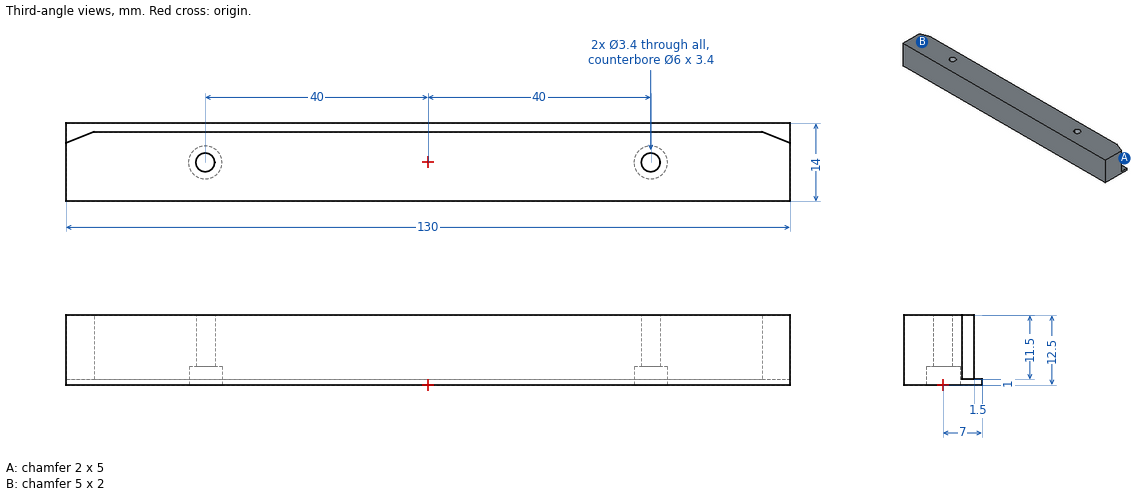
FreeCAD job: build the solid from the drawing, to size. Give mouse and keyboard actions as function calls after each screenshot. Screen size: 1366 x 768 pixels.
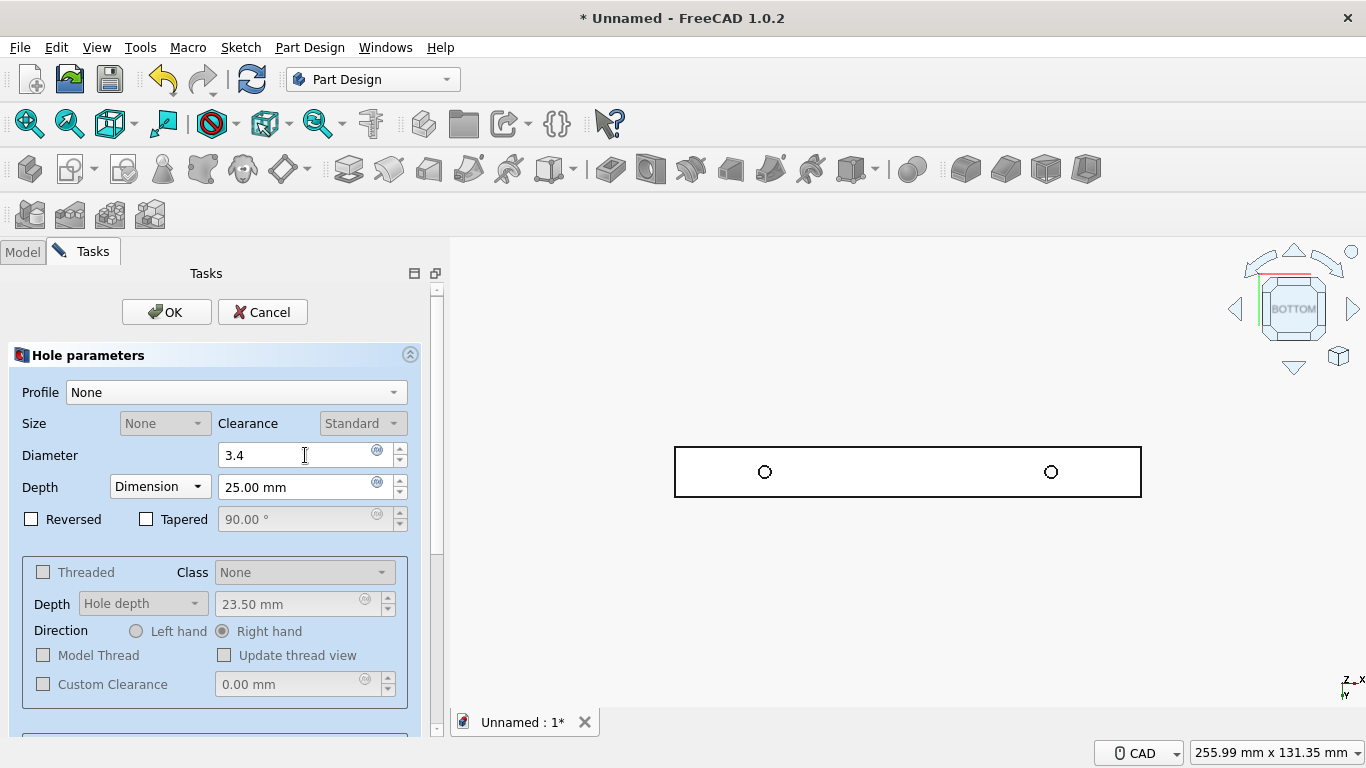
click(161, 486)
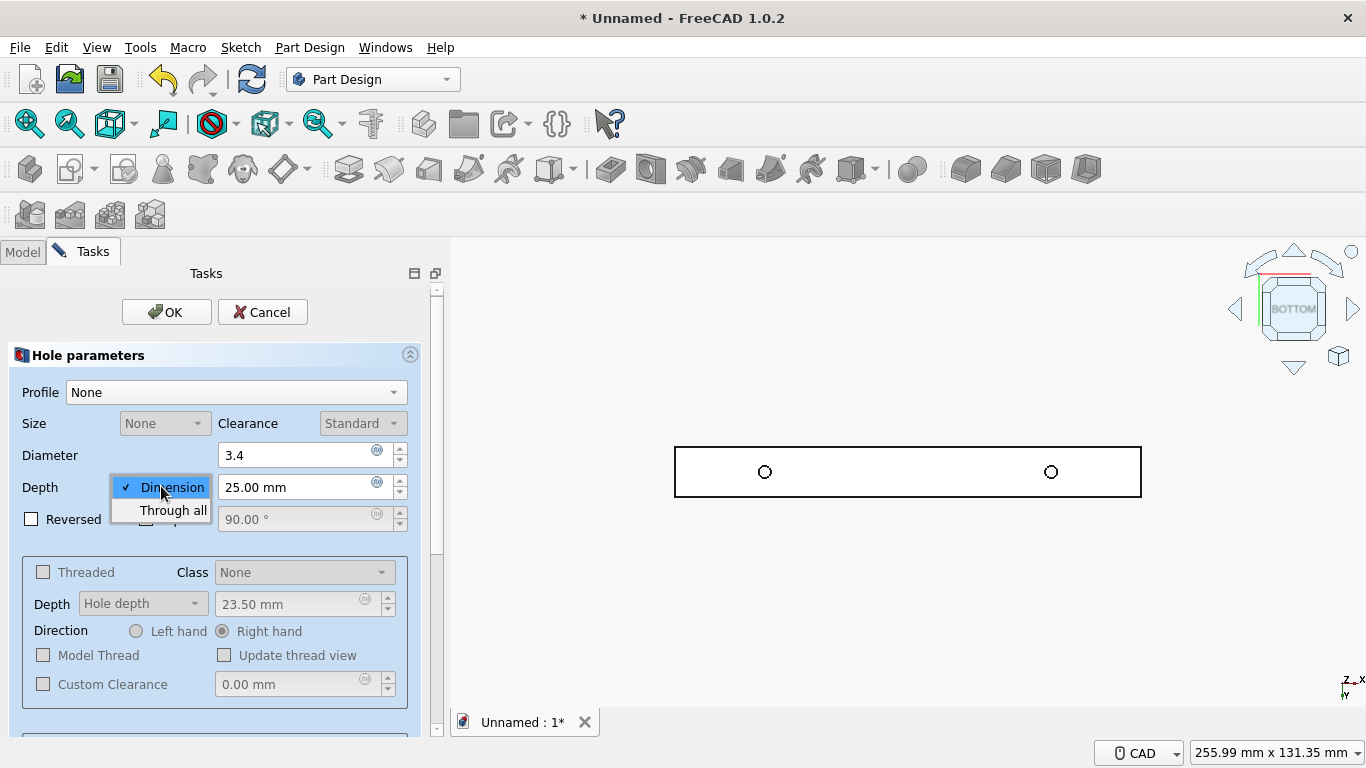
click(160, 510)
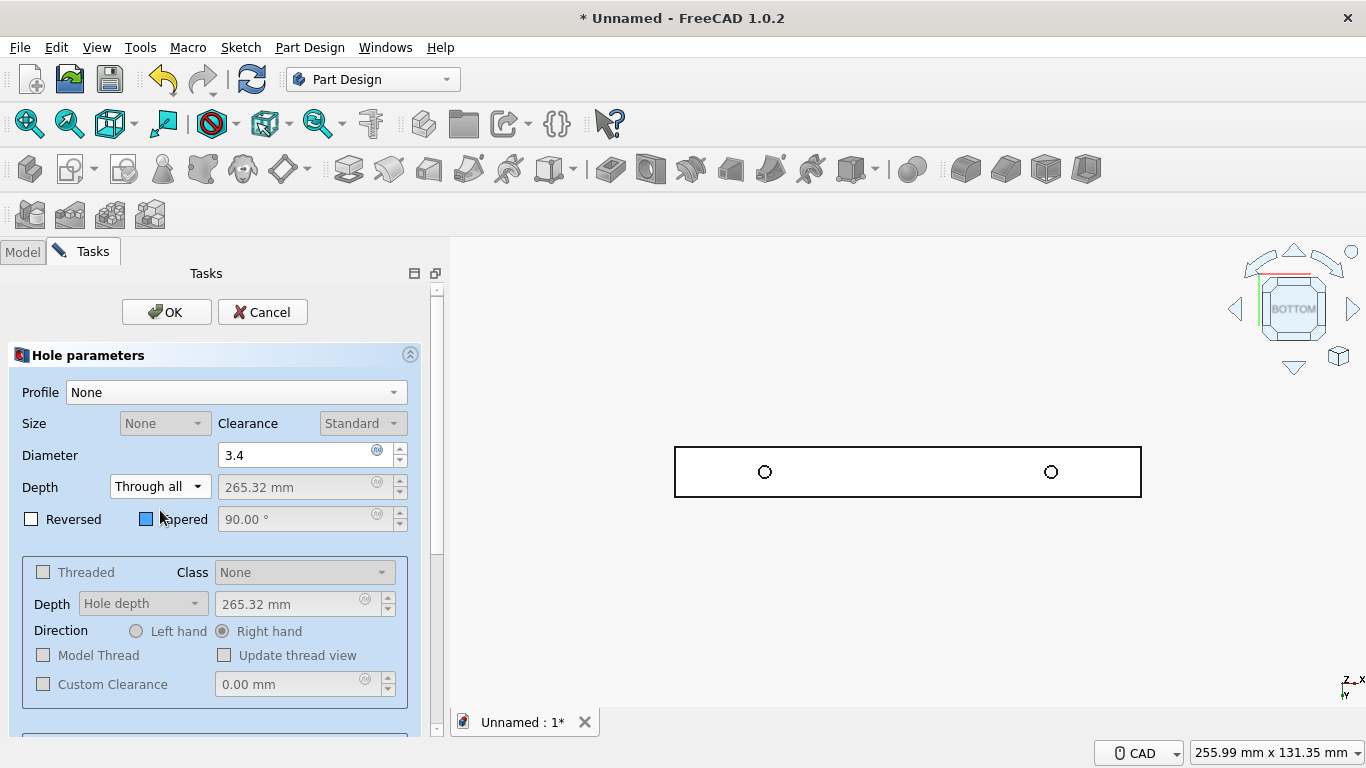
scroll(437, 510, down, 2)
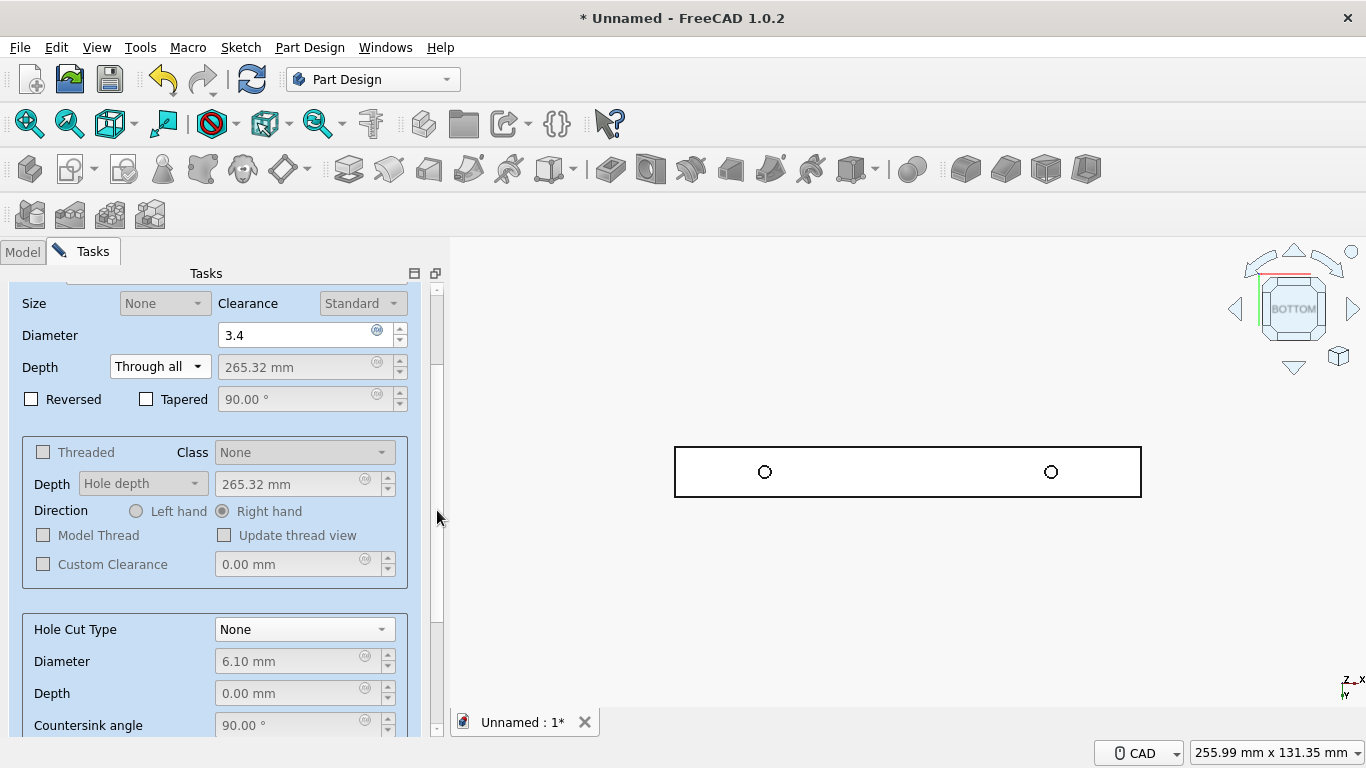
click(306, 630)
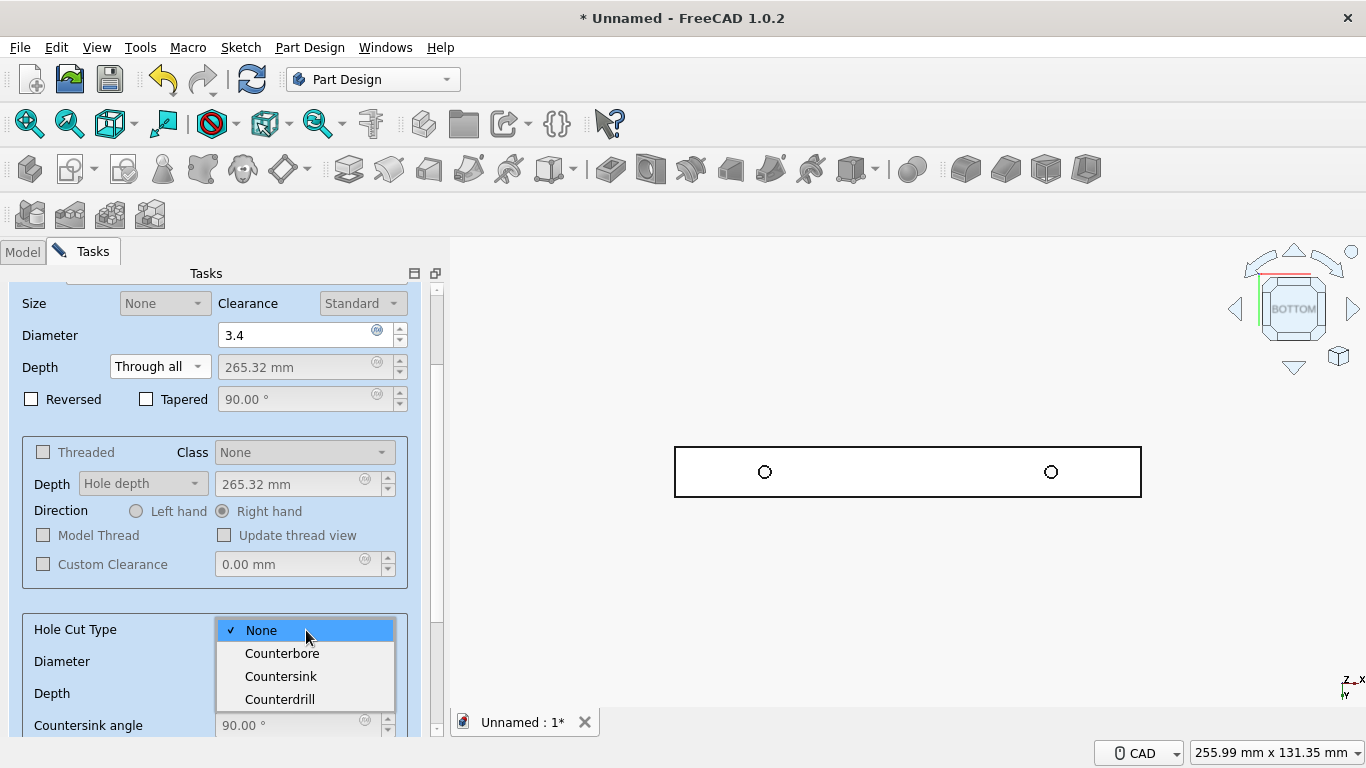
click(304, 654)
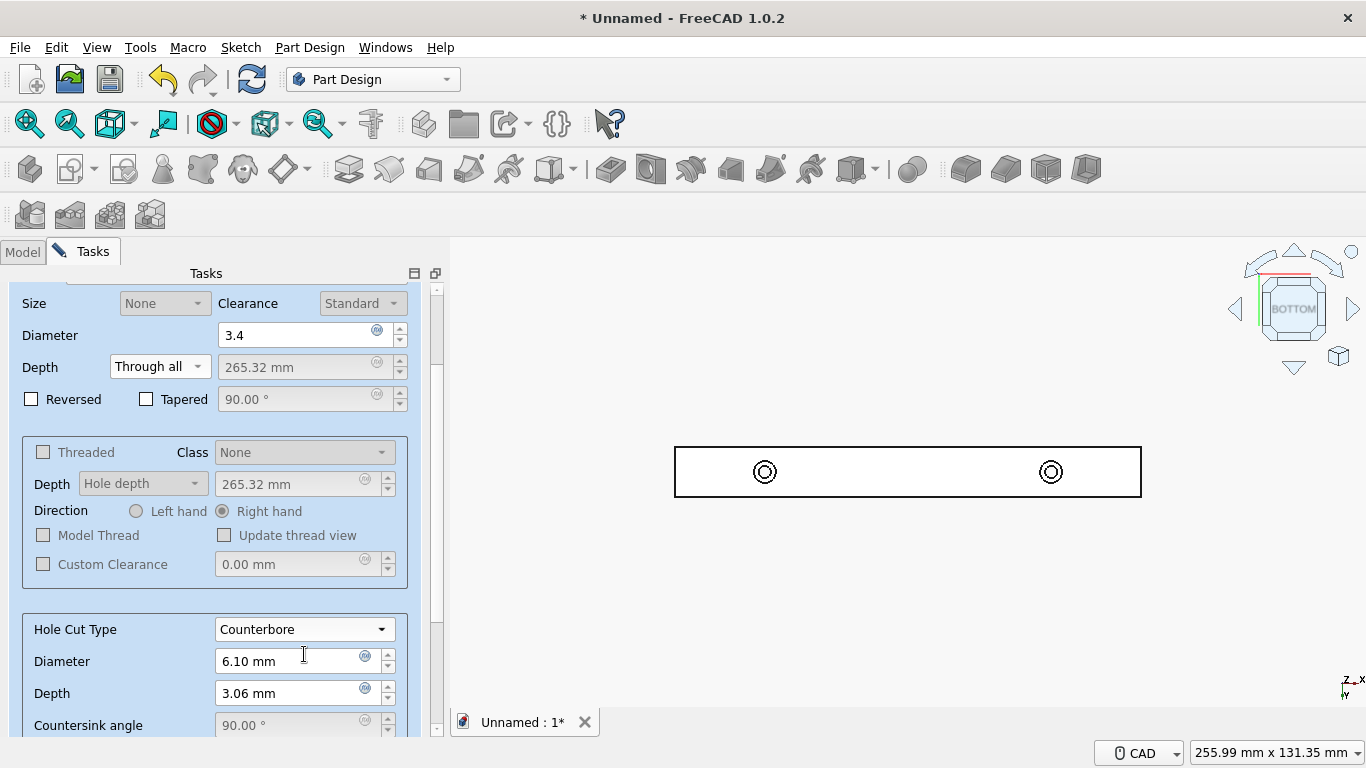
triple_click(298, 661)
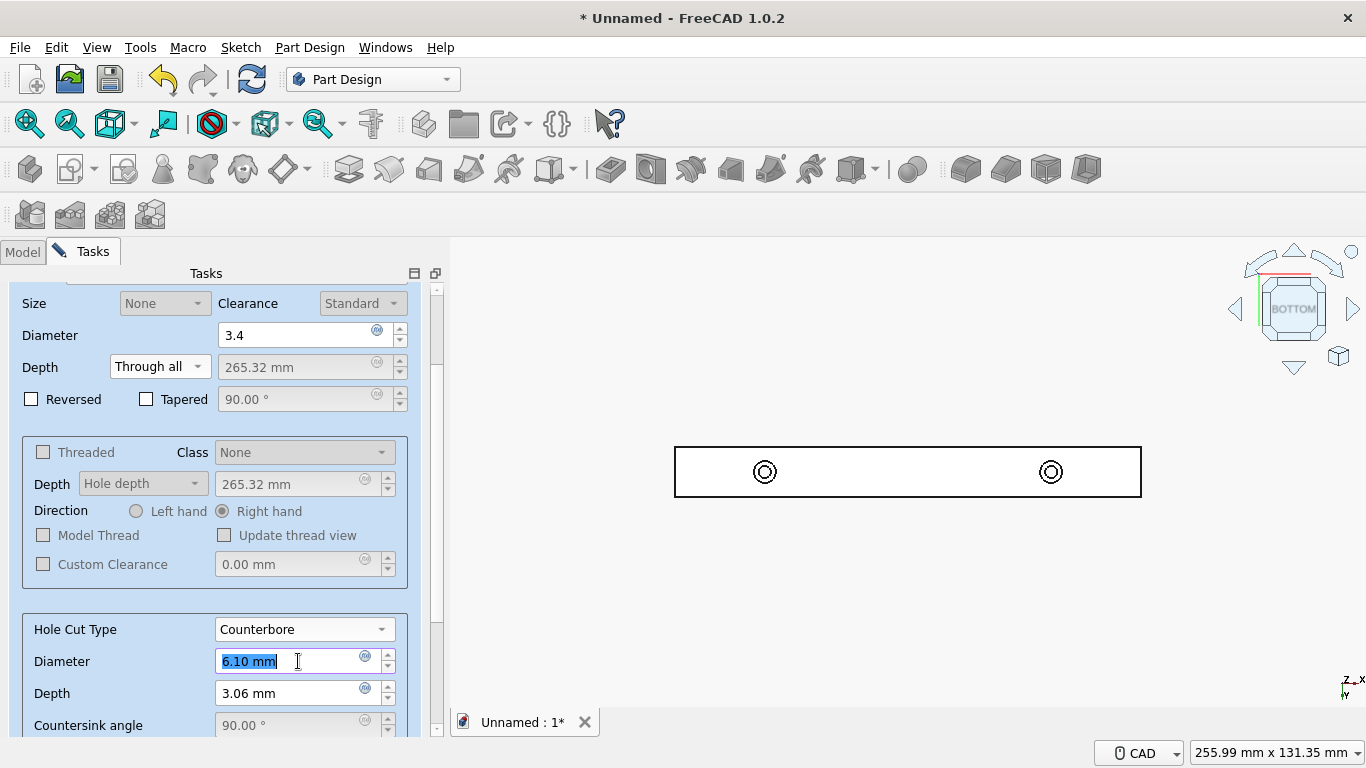
text(6)
key(Tab)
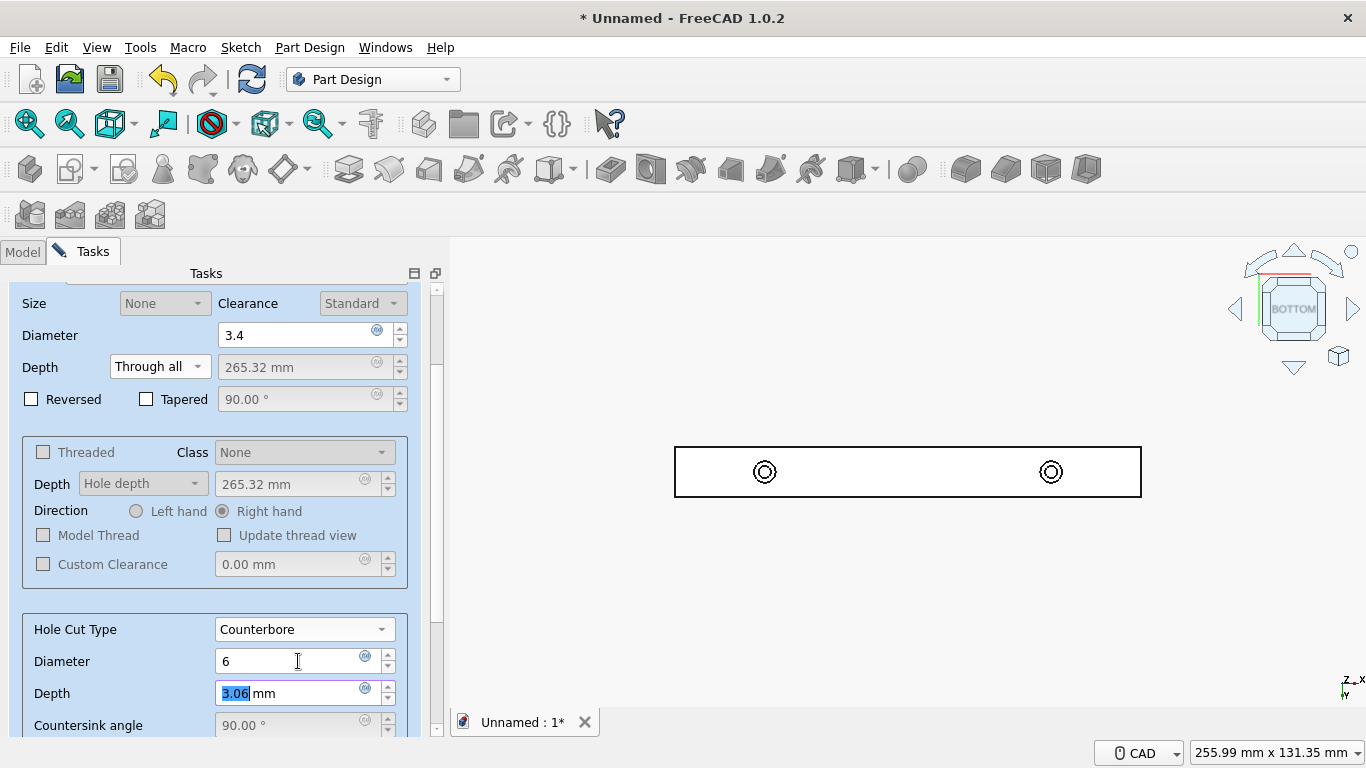
text(3.4)
key(Tab)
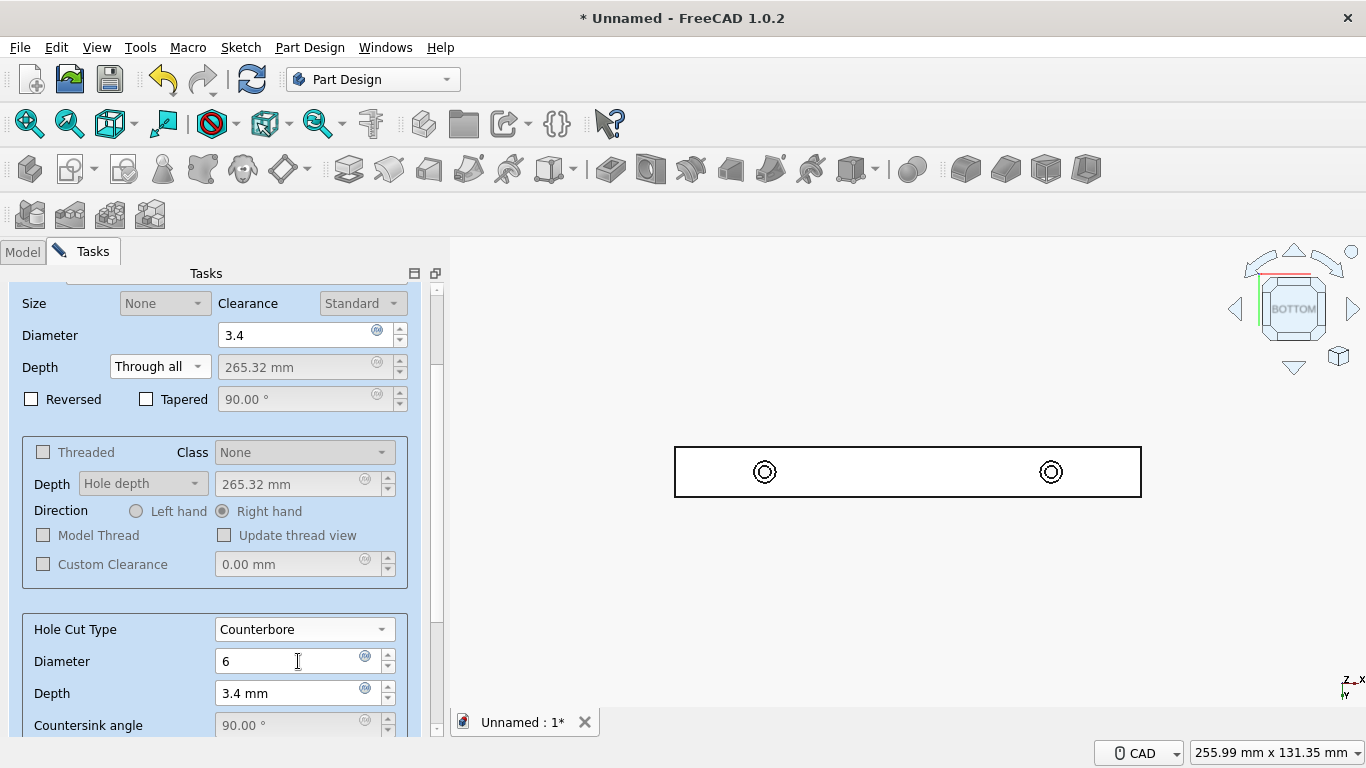
scroll(437, 510, up, 3)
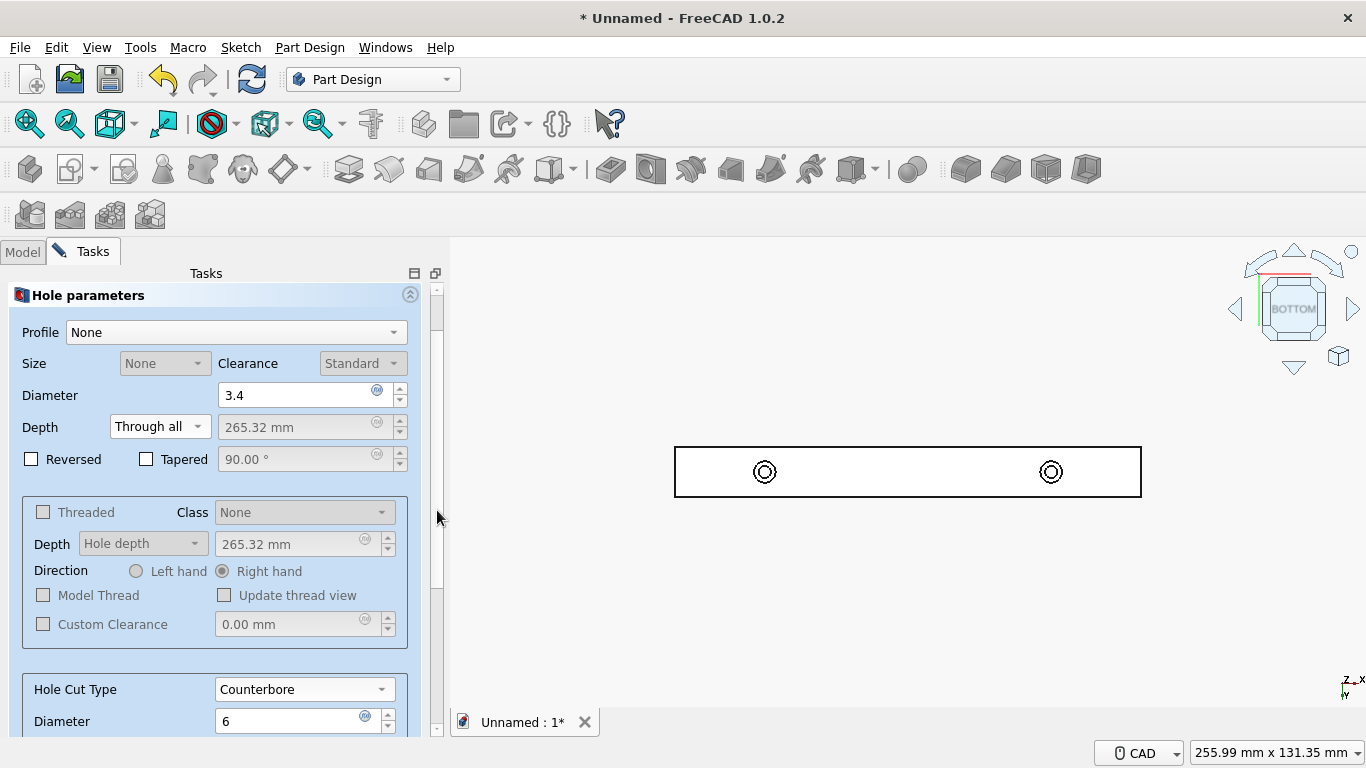
click(167, 312)